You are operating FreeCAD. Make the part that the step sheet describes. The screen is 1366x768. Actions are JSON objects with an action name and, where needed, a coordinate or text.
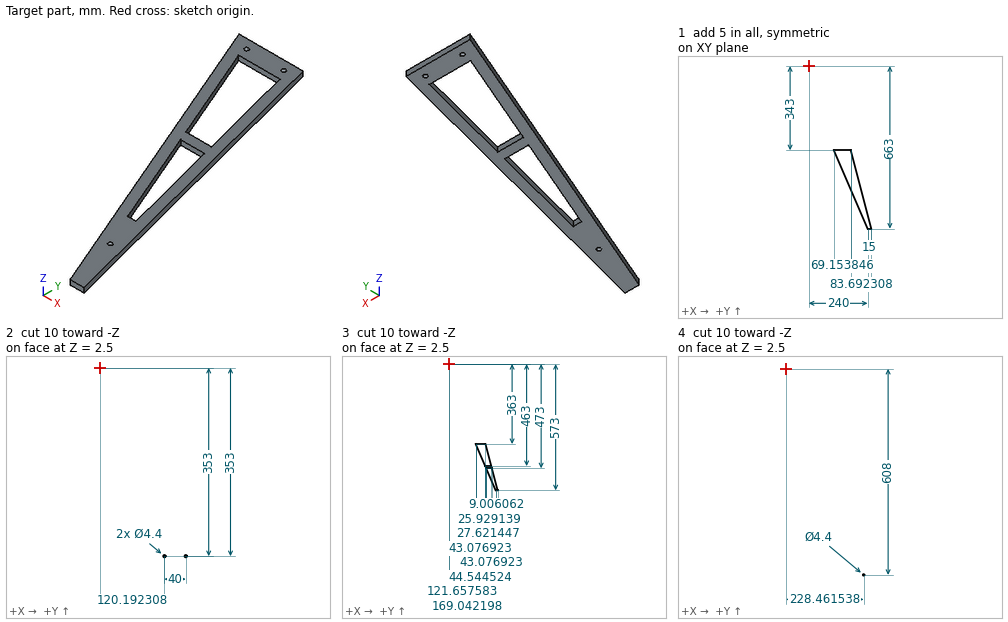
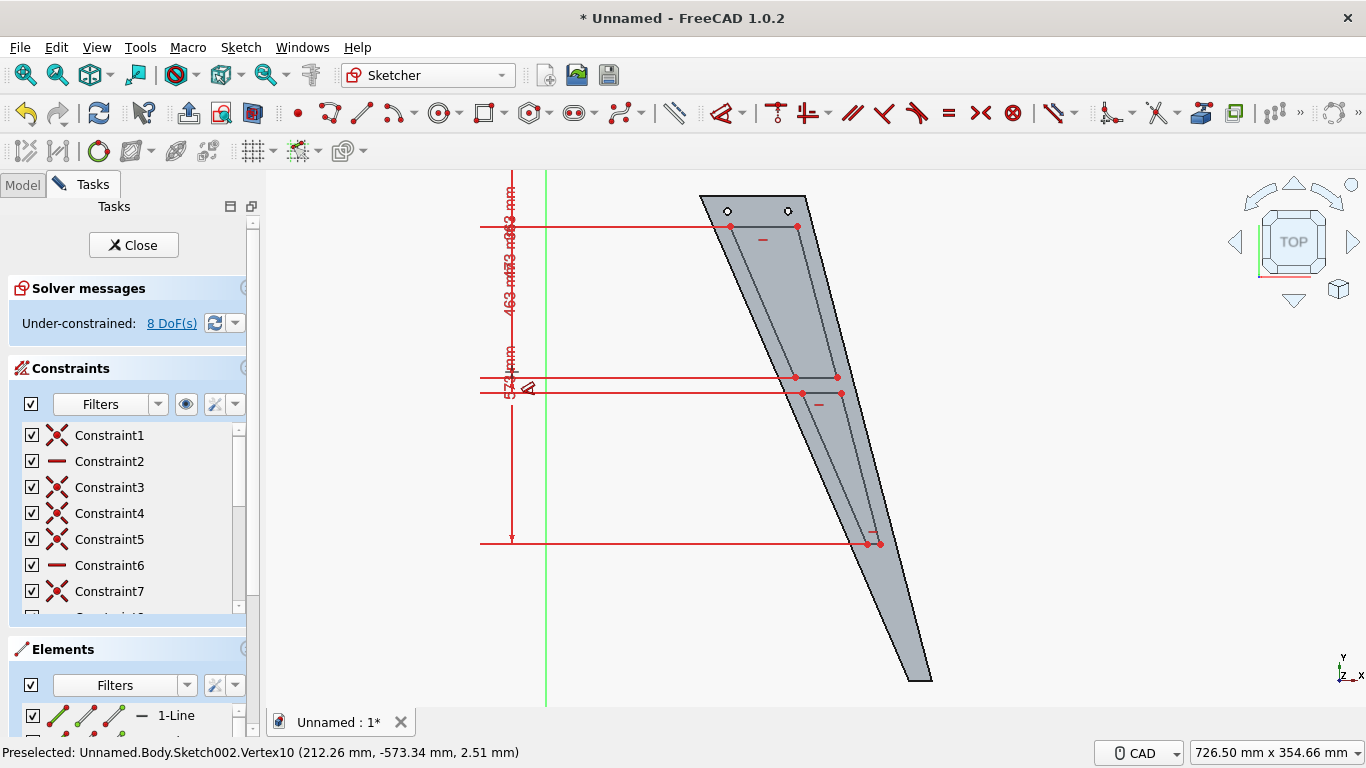
{"action": "scroll", "coordinate": [873, 544], "scroll_direction": "up", "scroll_amount": 6}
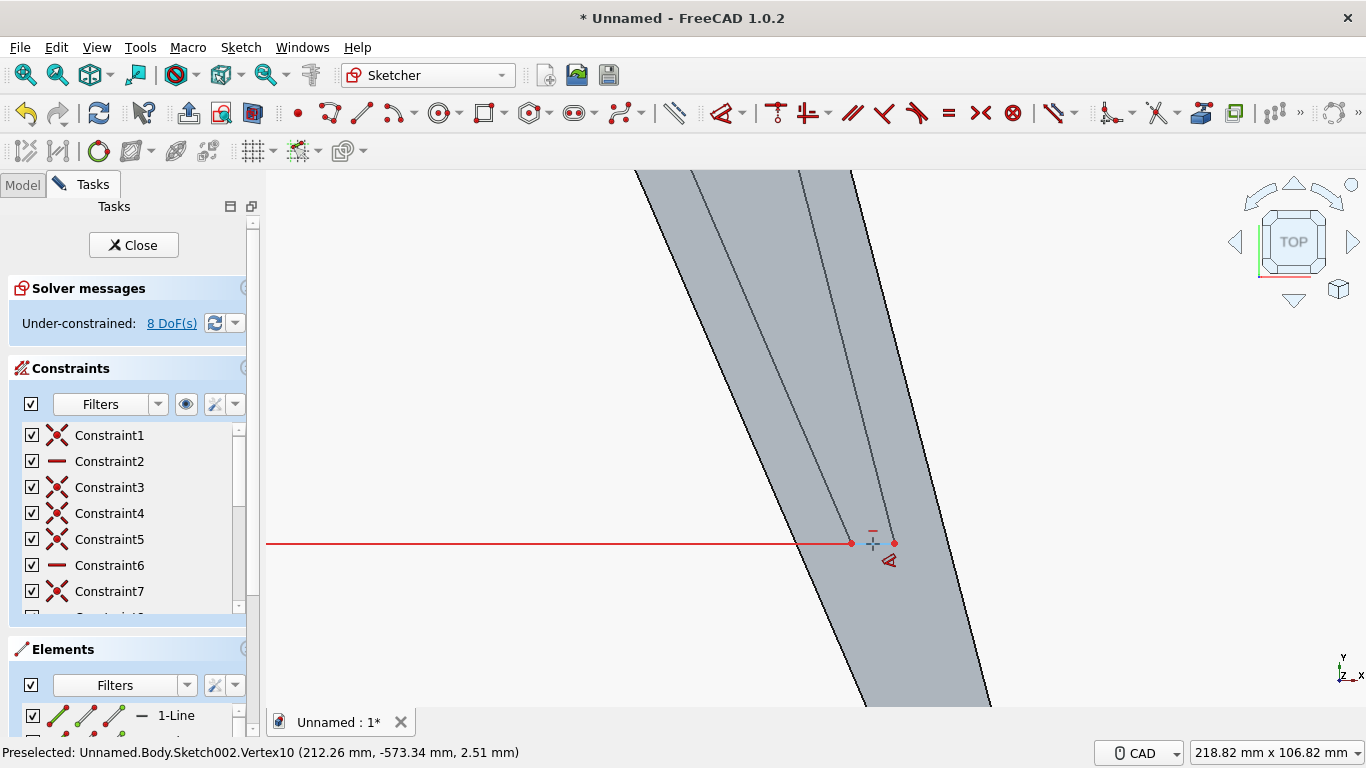
{"action": "left_click", "coordinate": [873, 544]}
{"action": "left_click", "coordinate": [873, 578]}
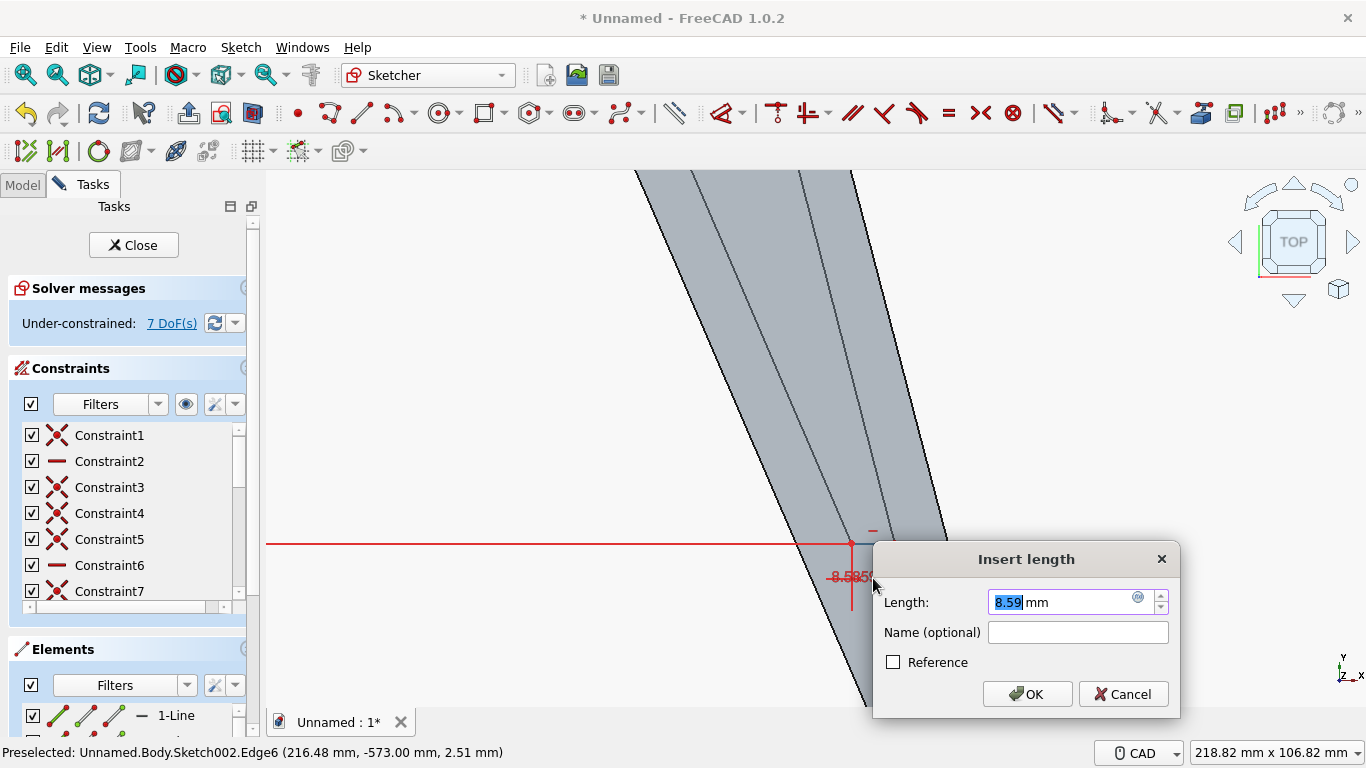
{"action": "type", "text": "9.006062"}
{"action": "key", "text": "Return"}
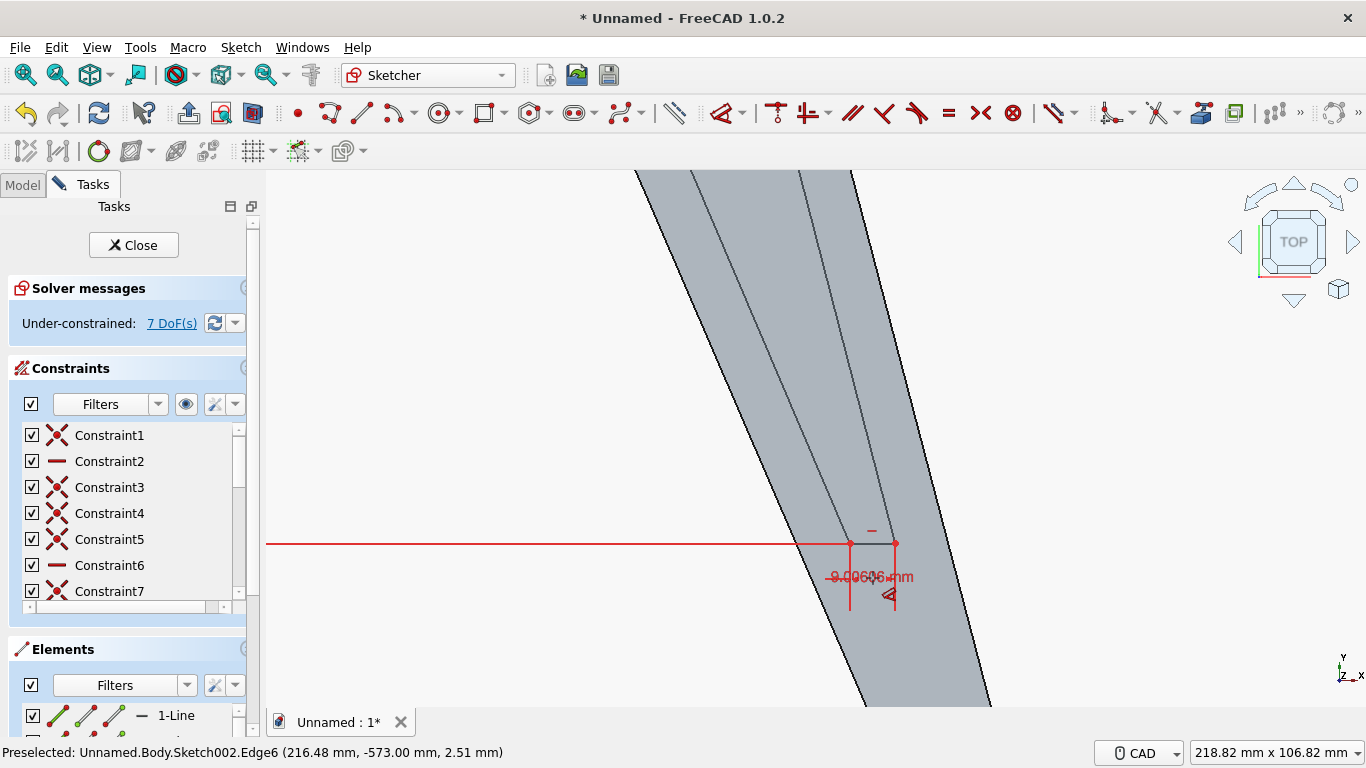
{"action": "scroll", "coordinate": [791, 621], "scroll_direction": "down", "scroll_amount": 6}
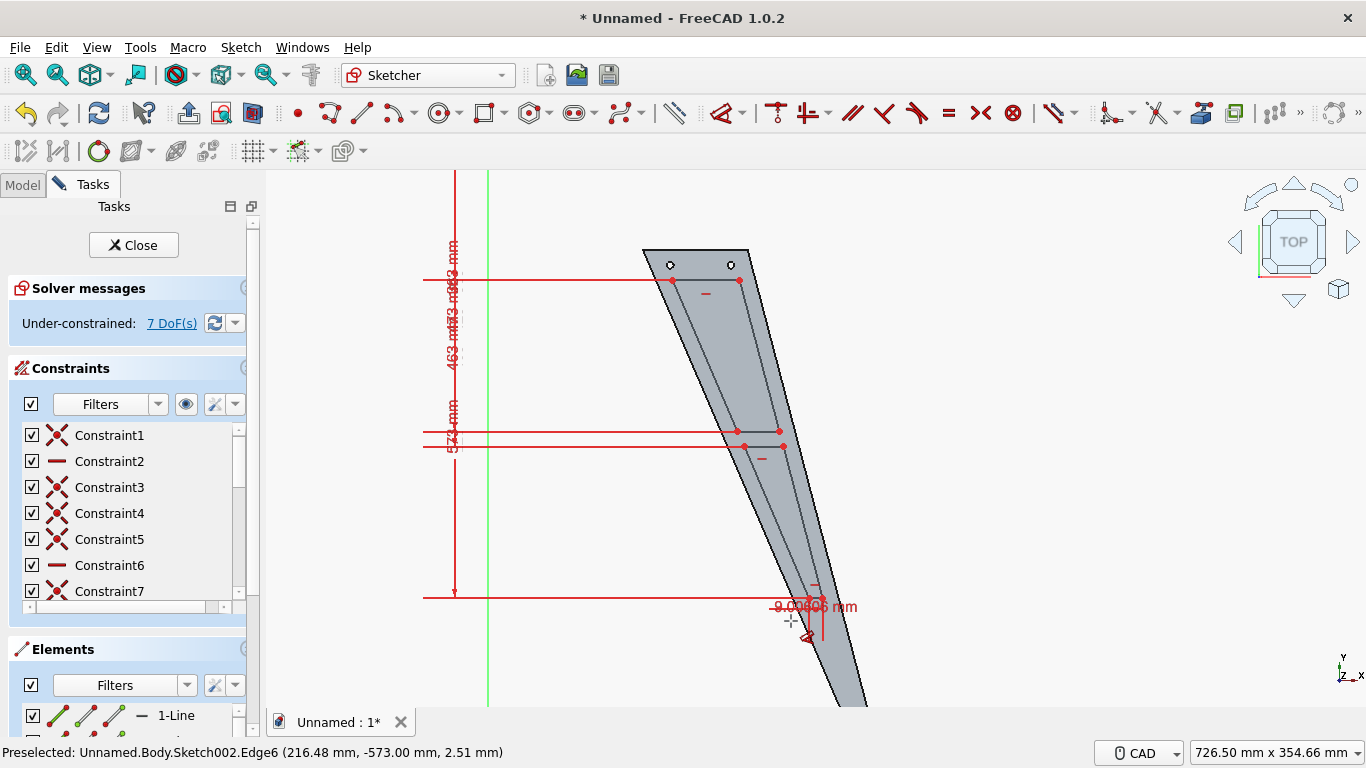
{"action": "left_click", "coordinate": [750, 432]}
{"action": "left_click", "coordinate": [749, 398]}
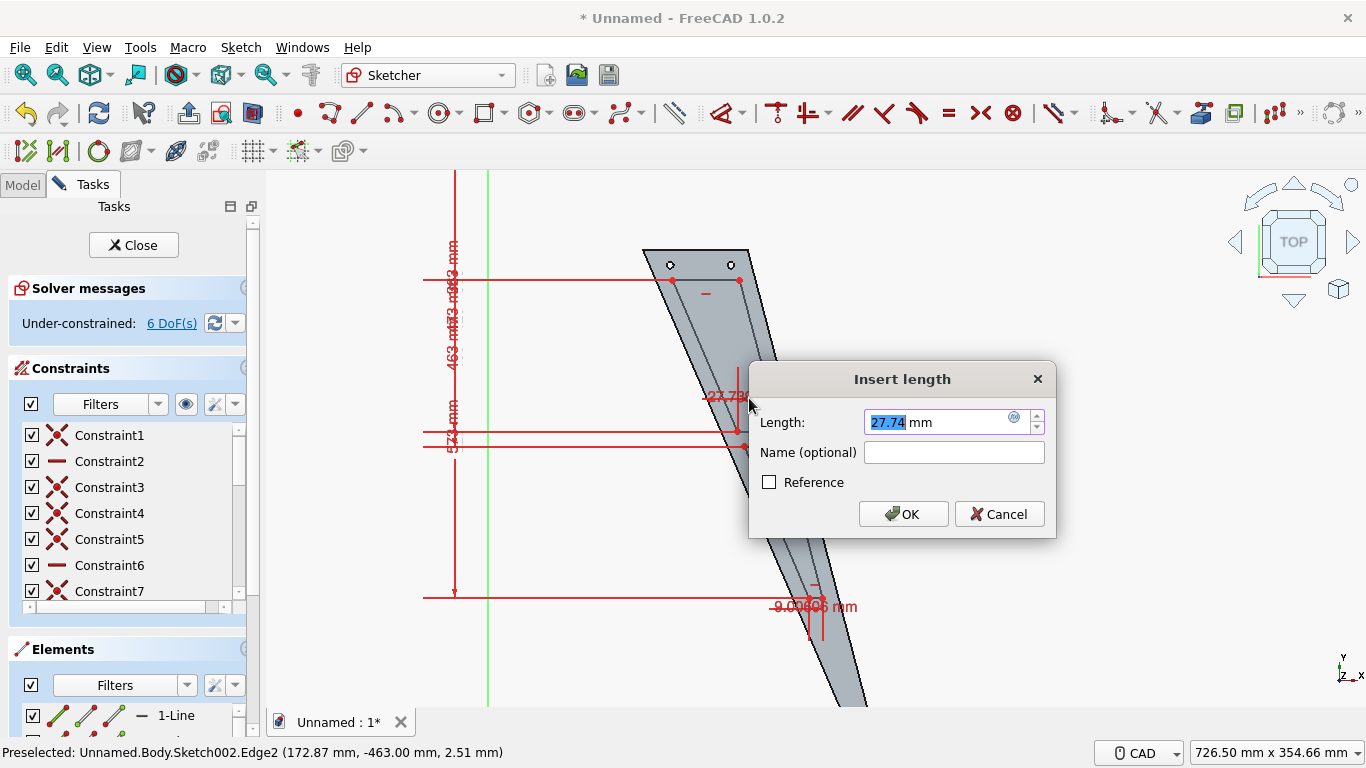
{"action": "type", "text": "27.621447"}
{"action": "key", "text": "Return"}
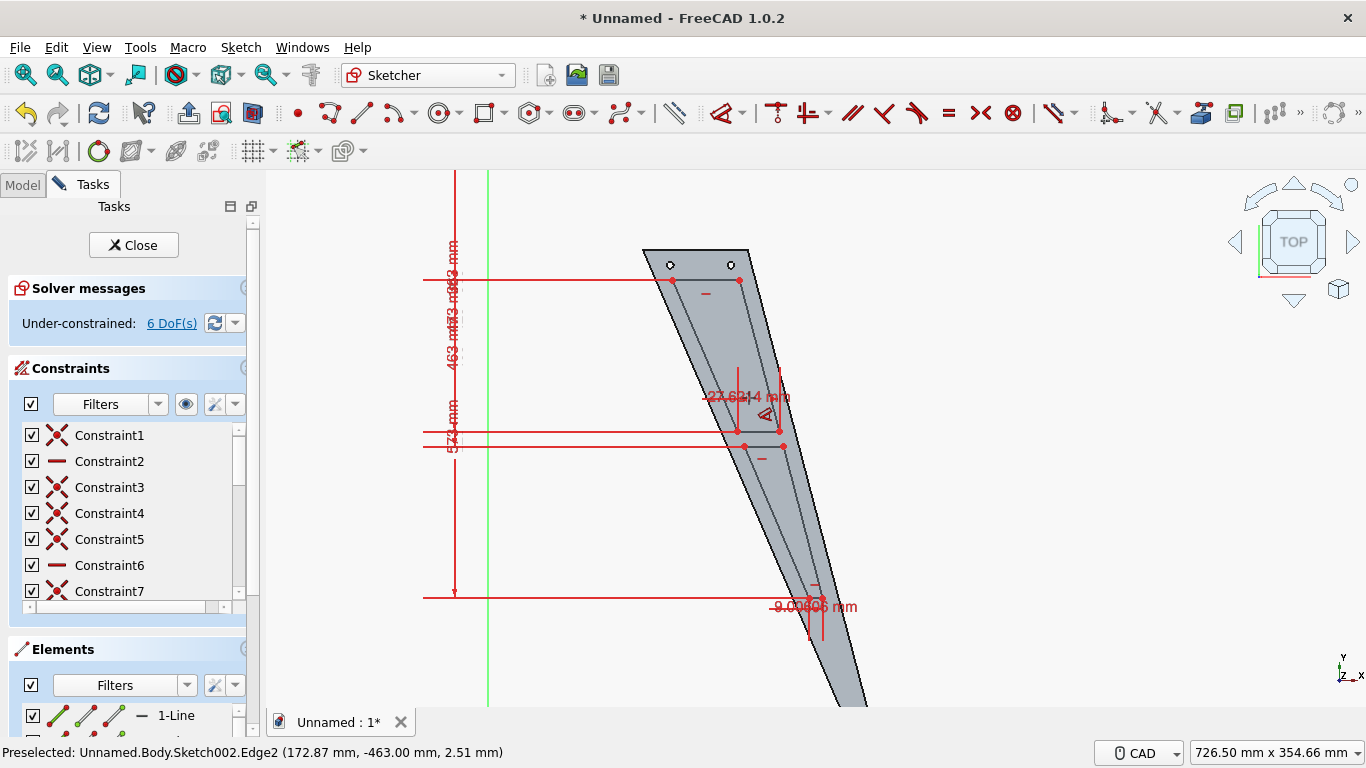
{"action": "left_click", "coordinate": [720, 280]}
{"action": "left_click", "coordinate": [706, 246]}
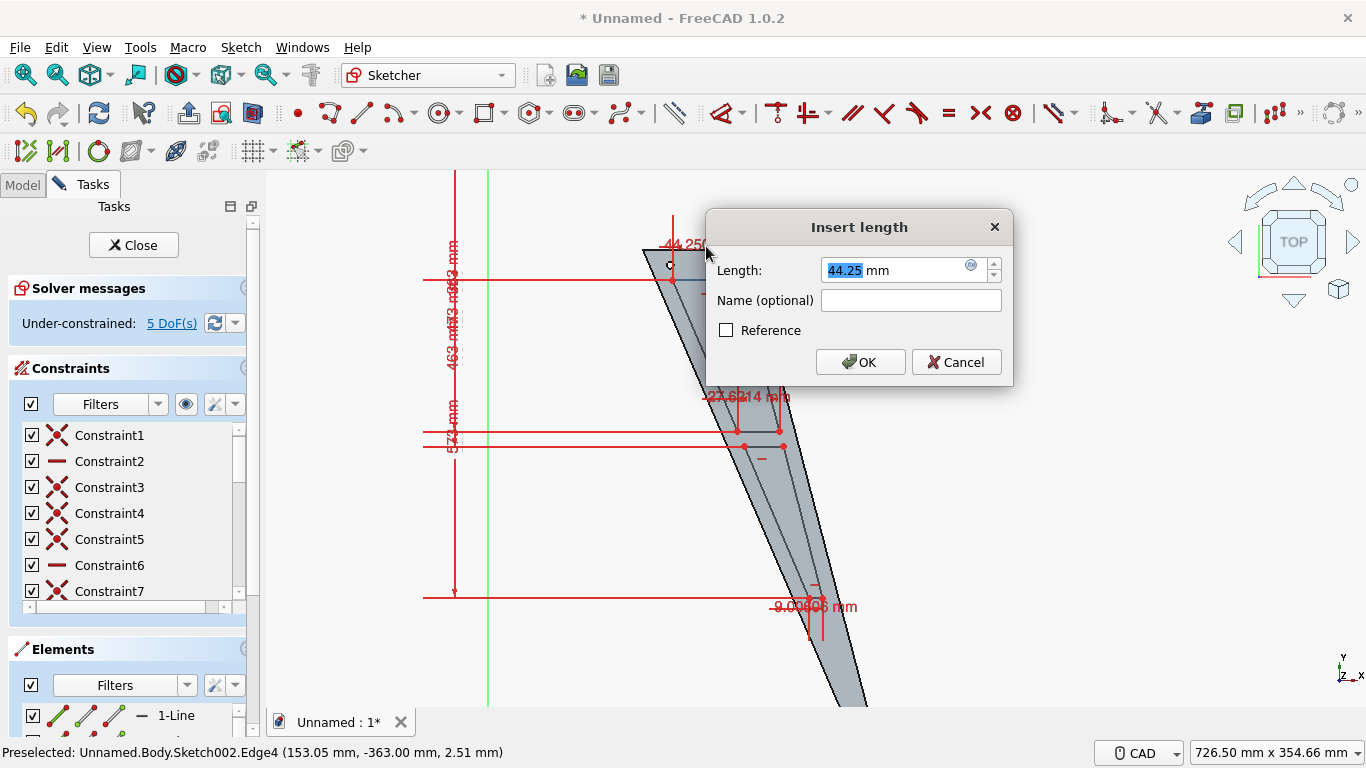
{"action": "type", "text": "44.544524"}
{"action": "key", "text": "Return"}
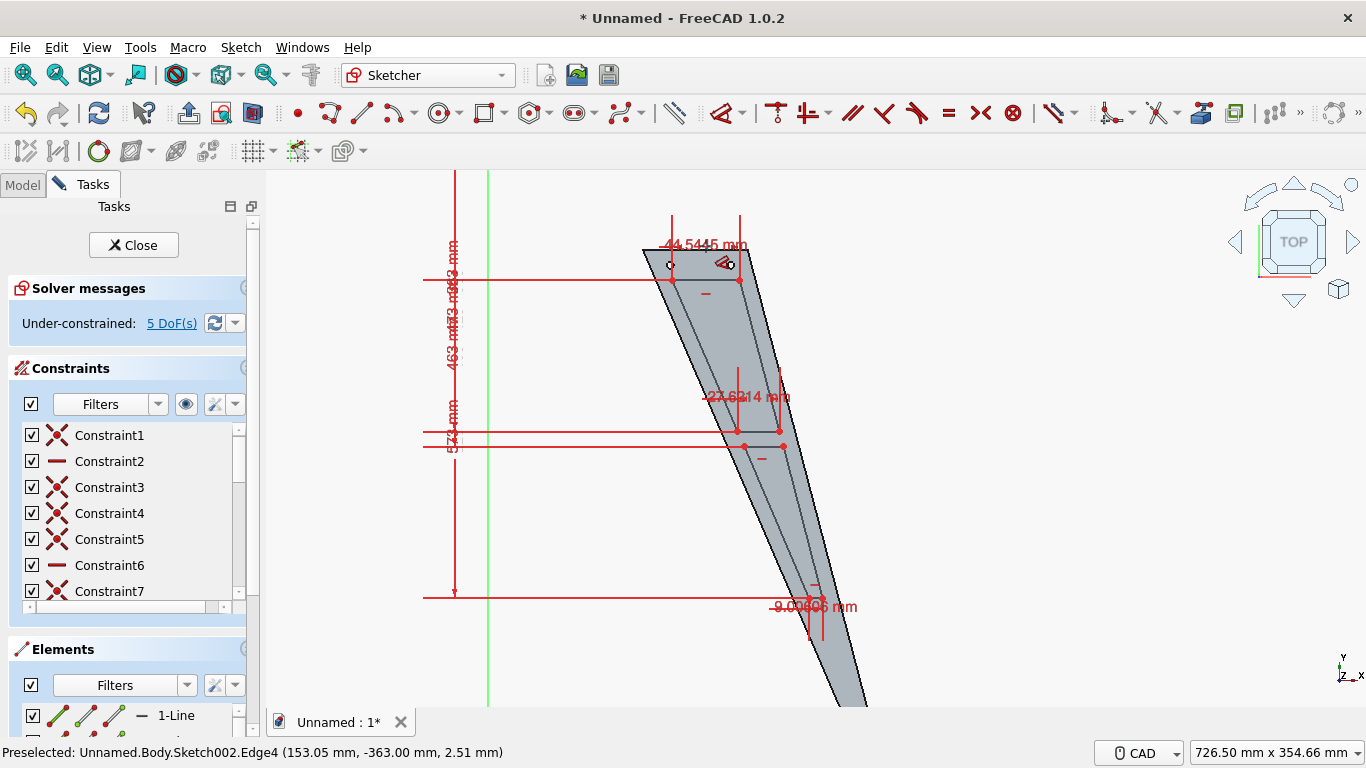
{"action": "left_click", "coordinate": [772, 447]}
{"action": "left_click", "coordinate": [778, 481]}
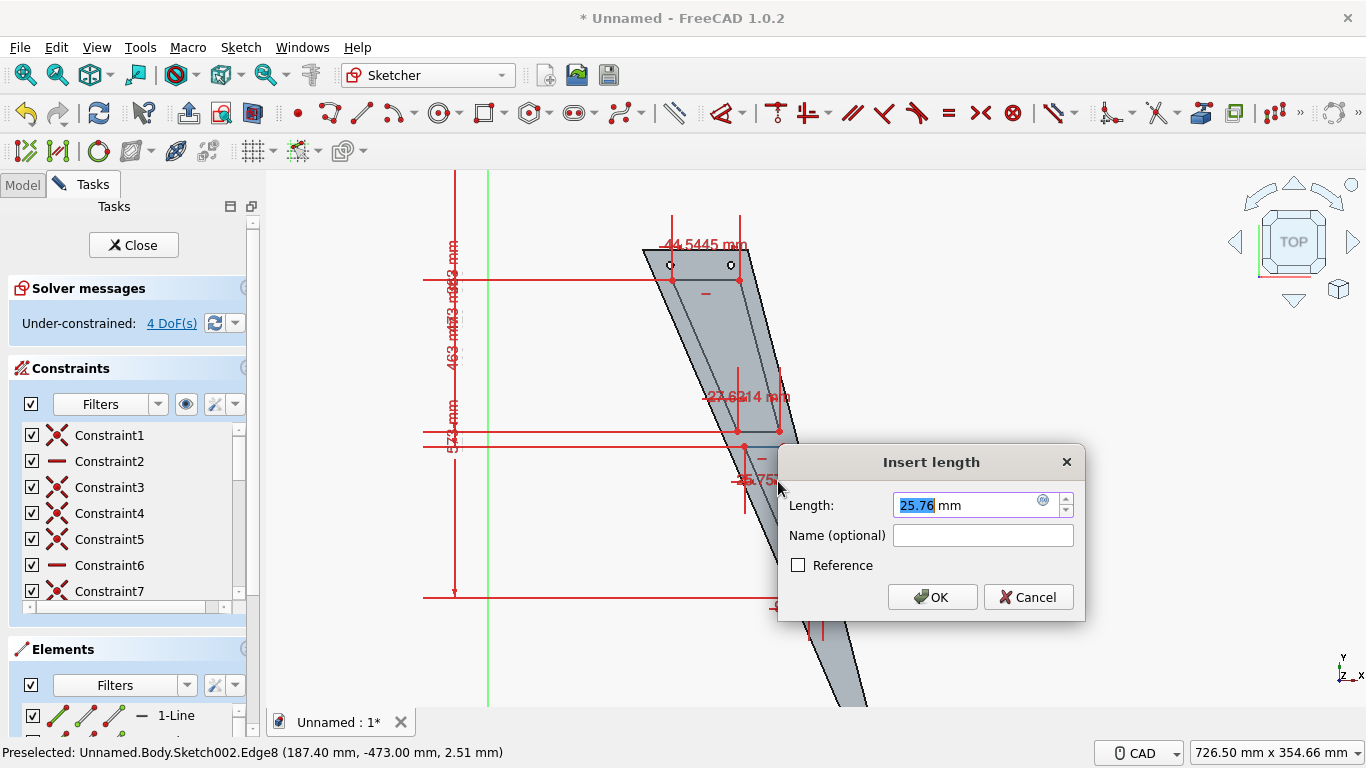
{"action": "type", "text": "25.929139"}
{"action": "key", "text": "Return"}